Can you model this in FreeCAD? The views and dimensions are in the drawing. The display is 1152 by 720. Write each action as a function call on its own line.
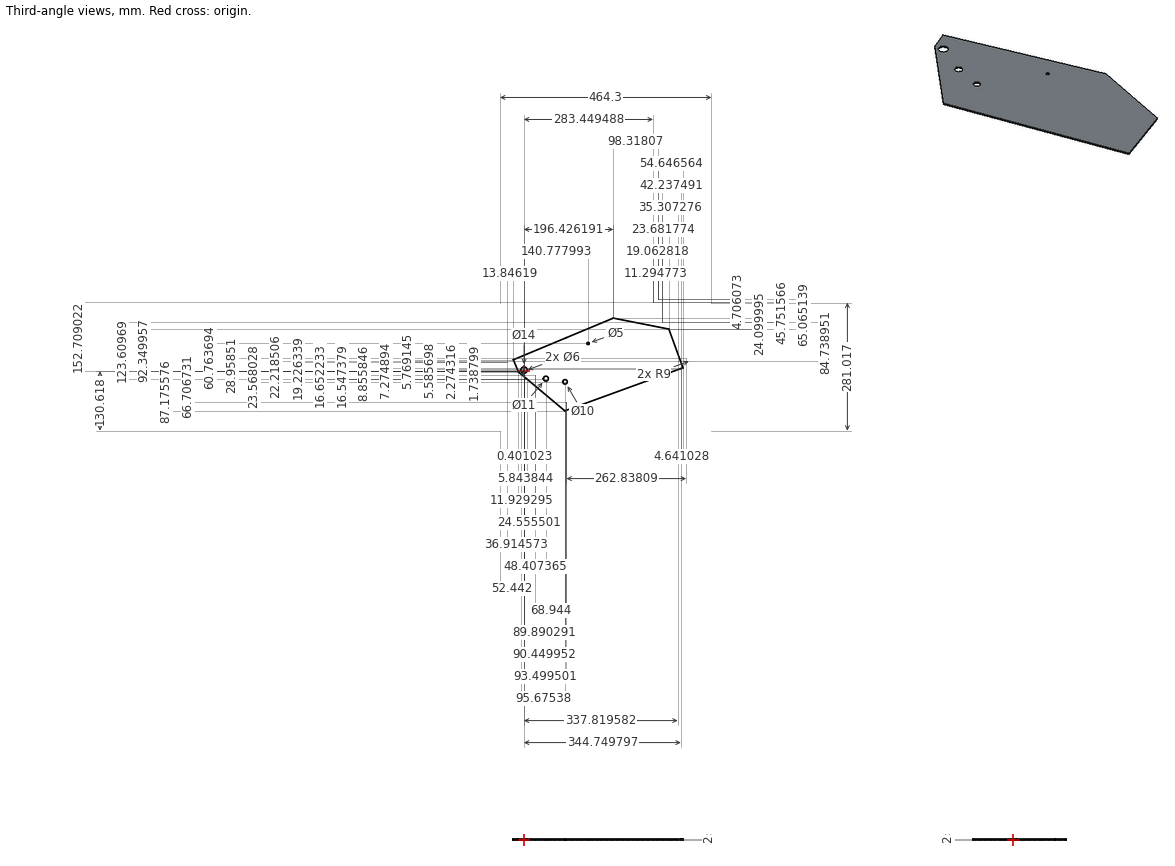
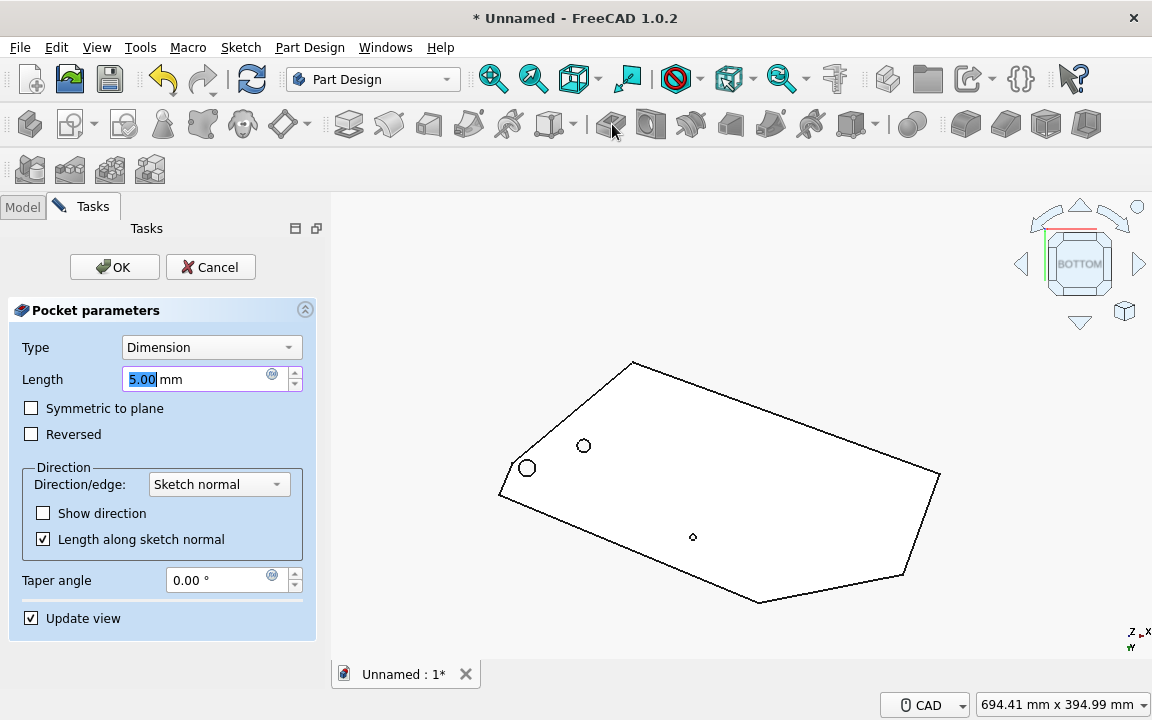
click(212, 348)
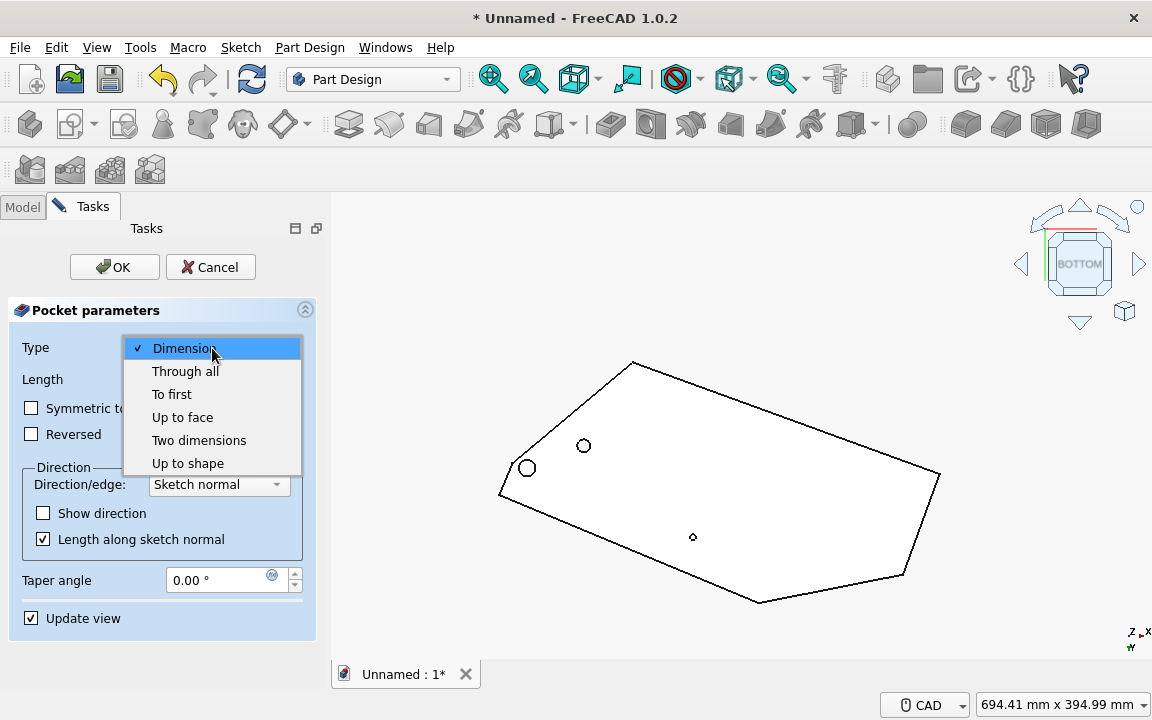
click(212, 372)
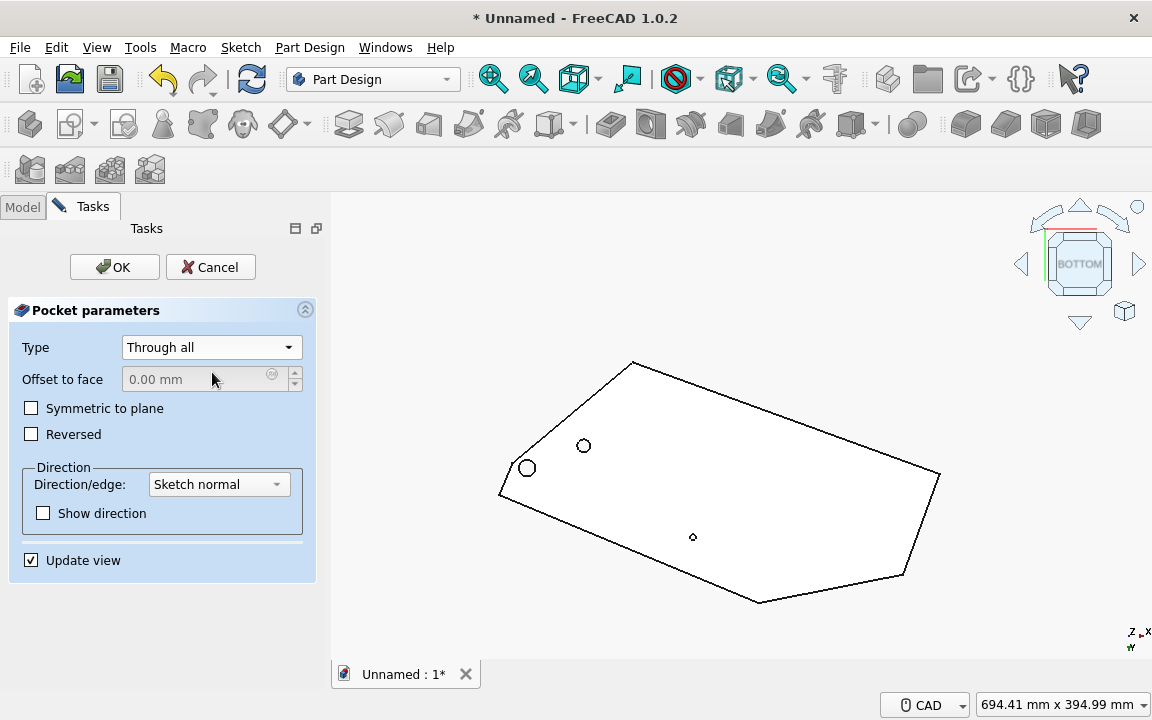
click(115, 267)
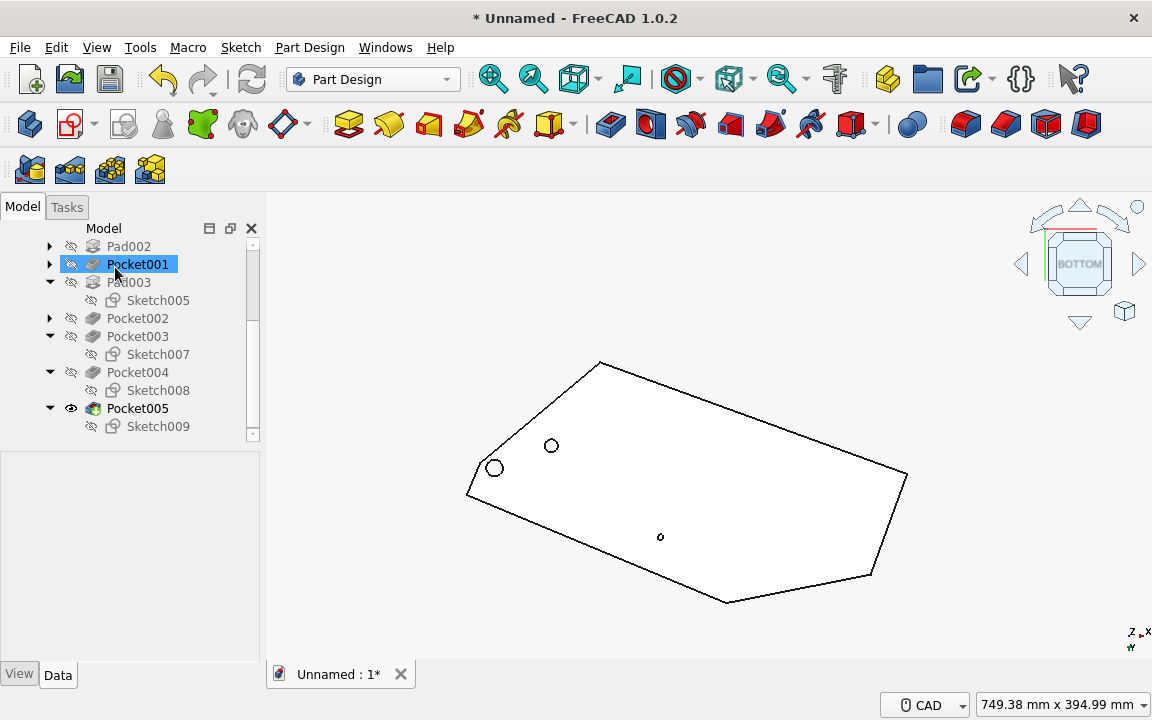
click(70, 124)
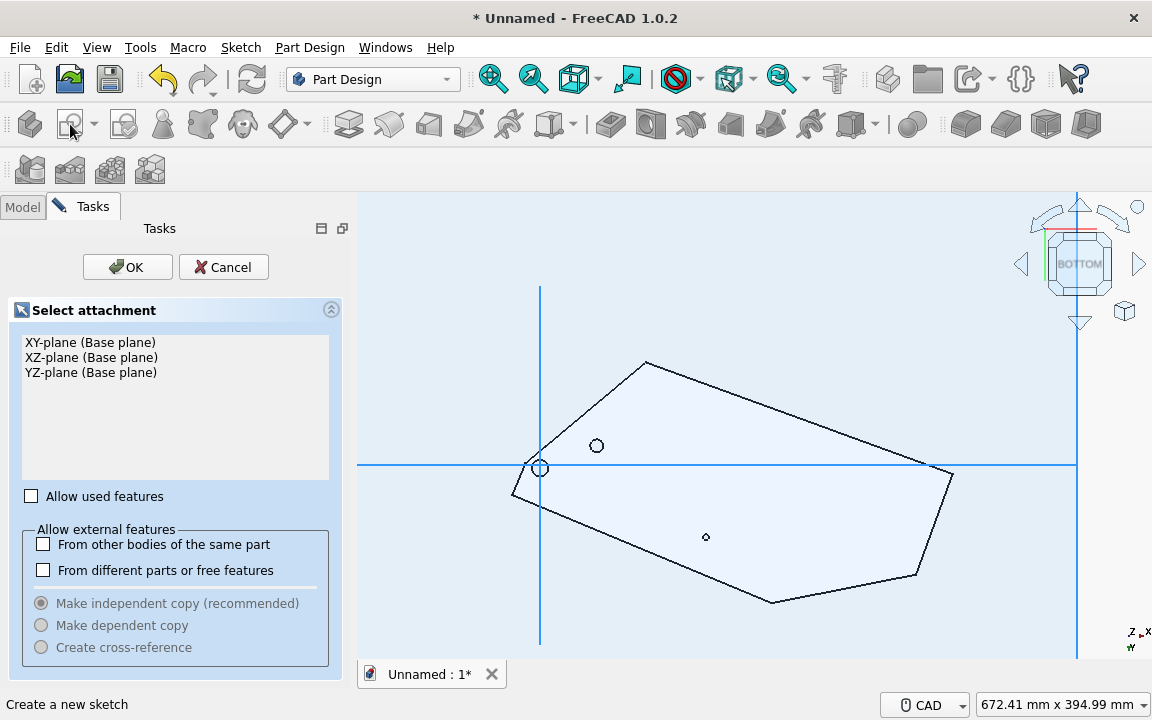
click(82, 342)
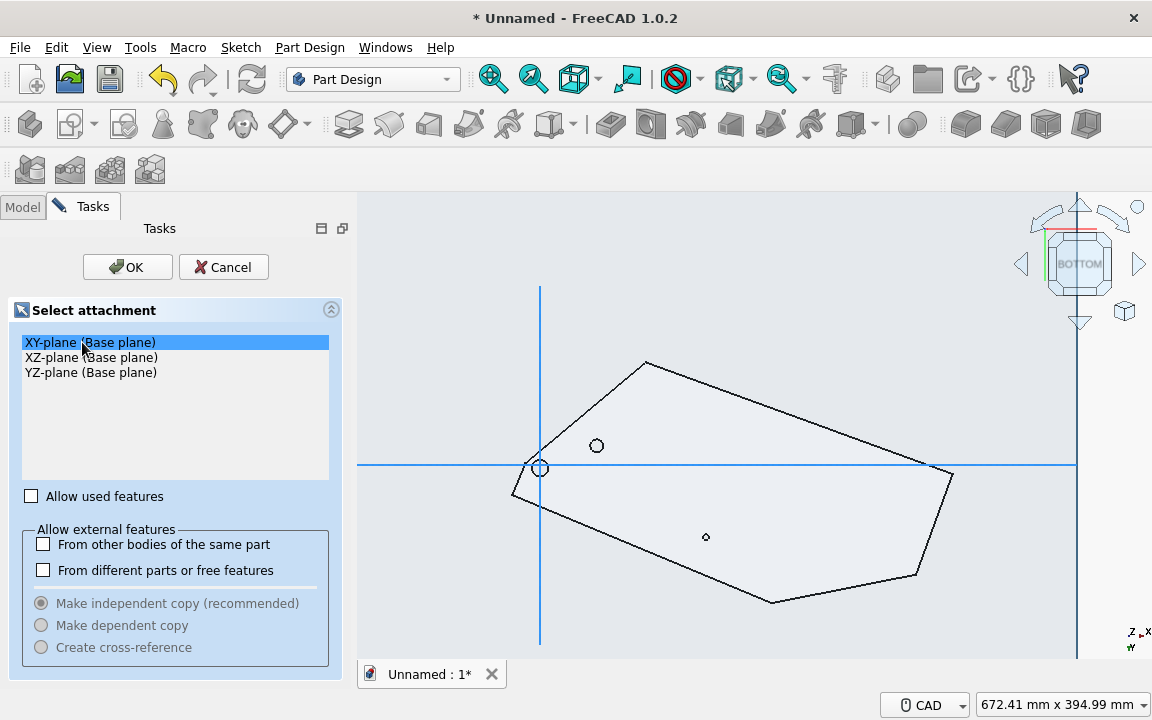
click(128, 267)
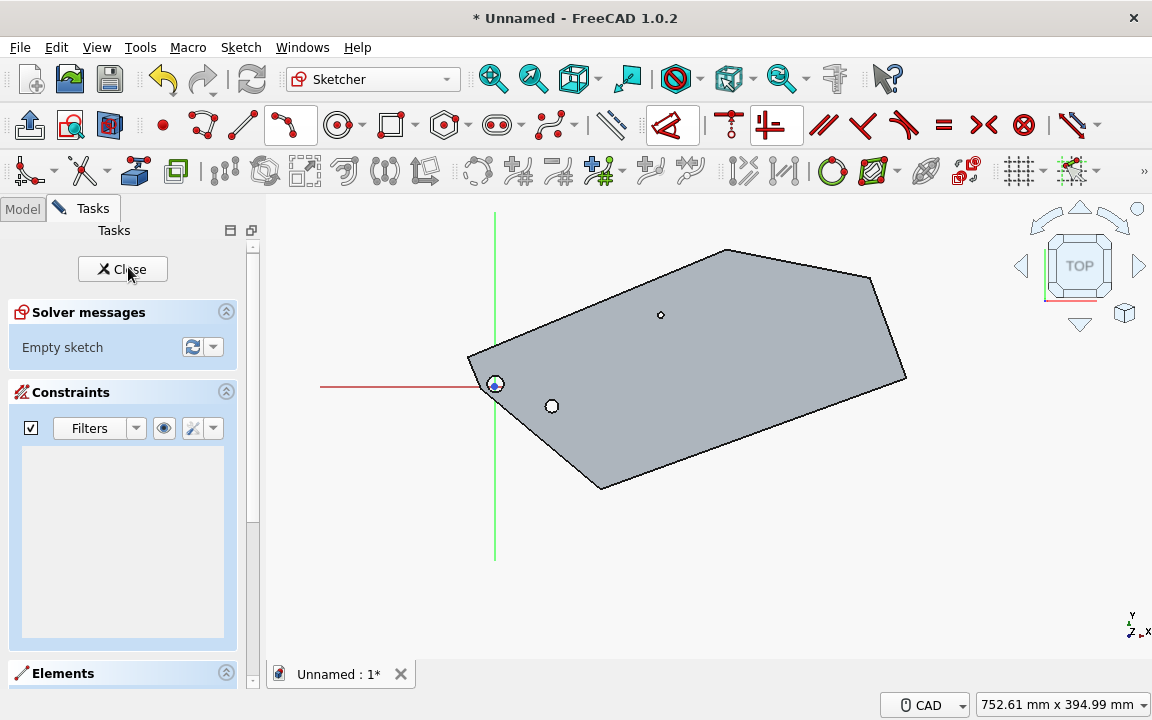
key(q)
key(s)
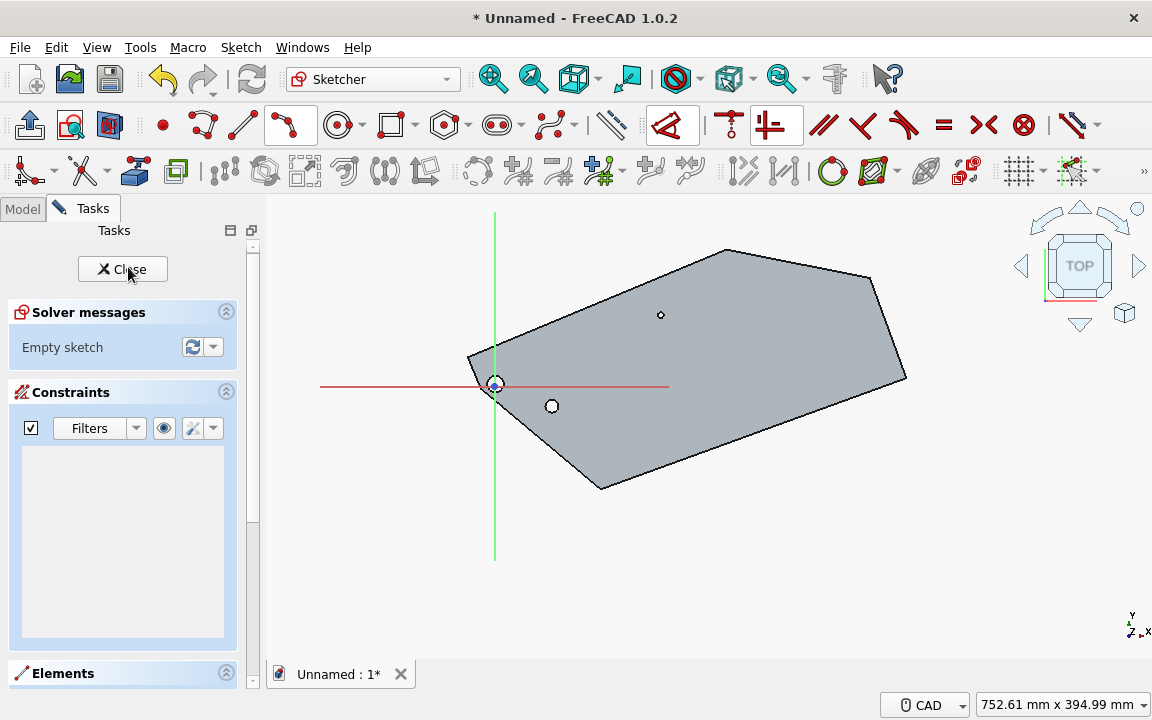
scroll(599, 414, up, 15)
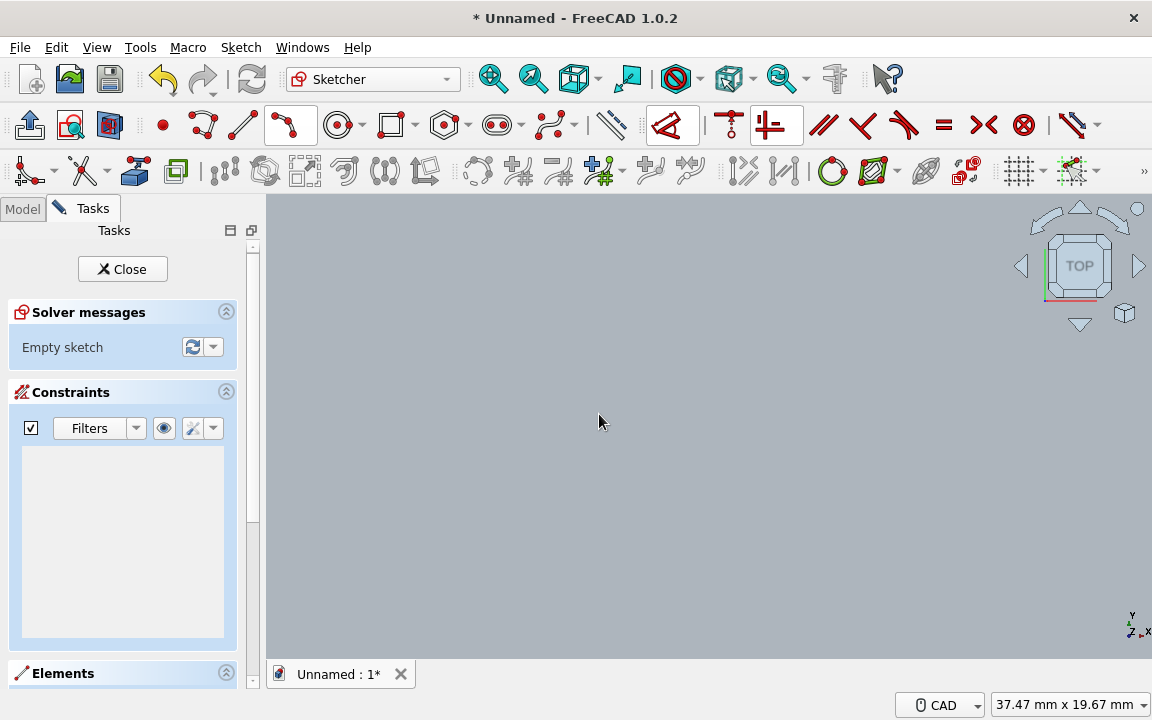
click(338, 126)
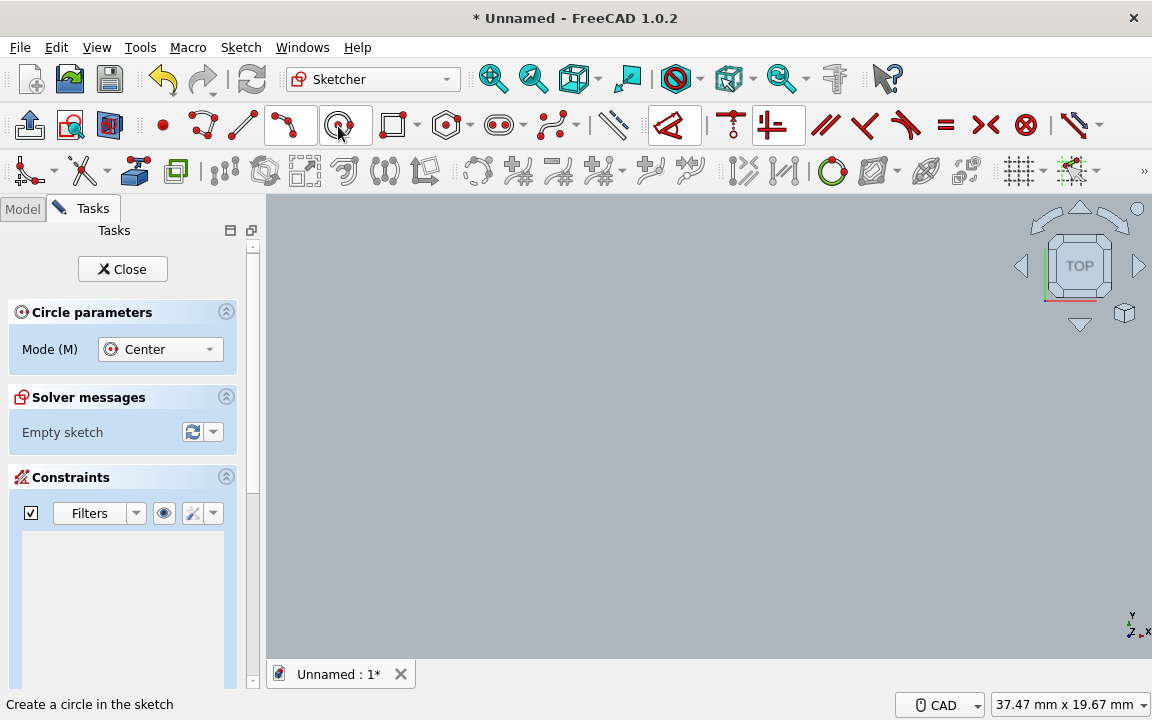
click(641, 414)
move(725, 331)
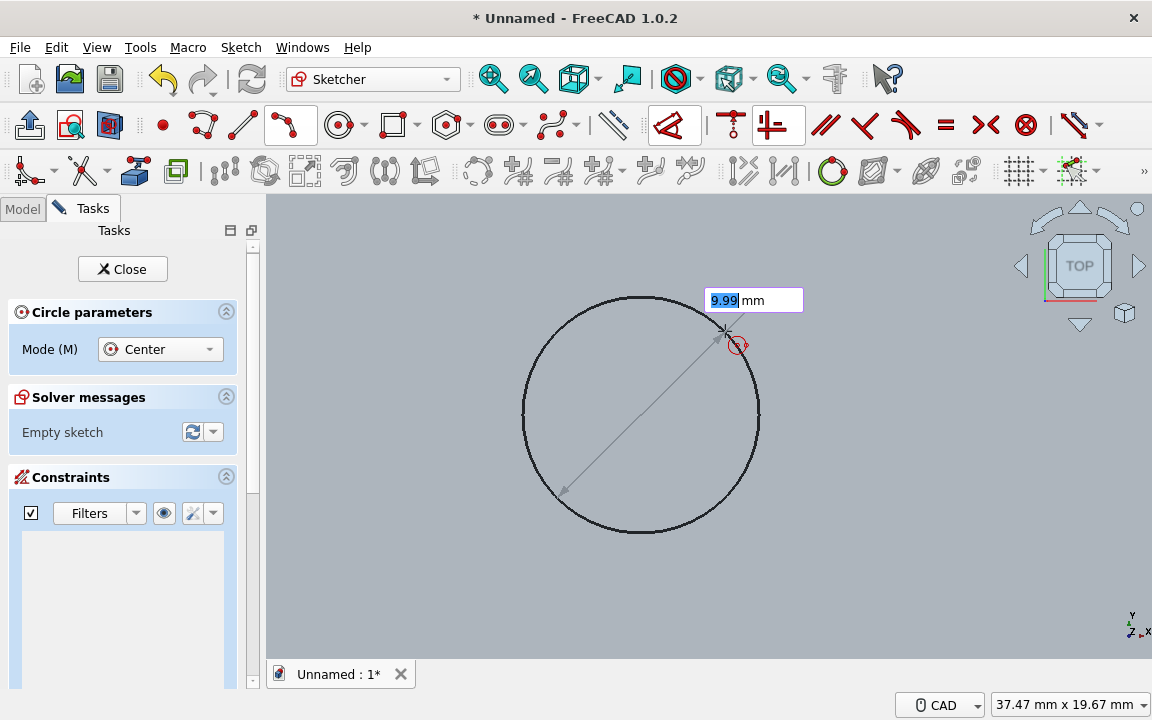
text(10)
key(Return)
key(Escape)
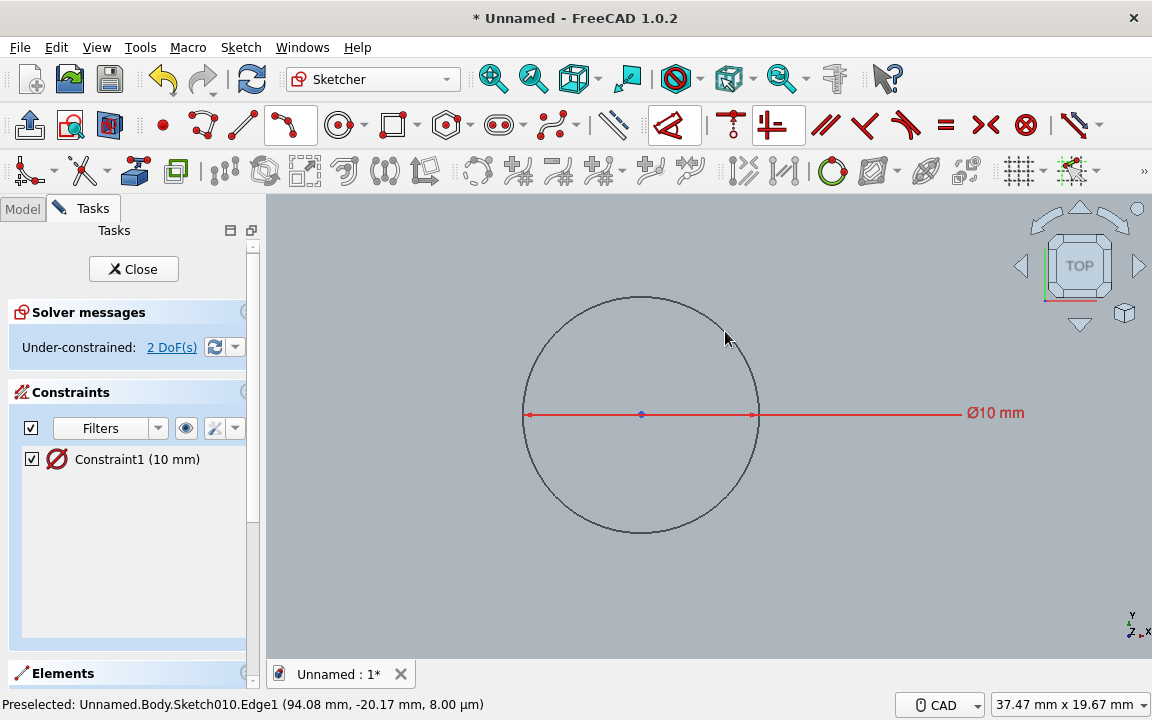
click(641, 415)